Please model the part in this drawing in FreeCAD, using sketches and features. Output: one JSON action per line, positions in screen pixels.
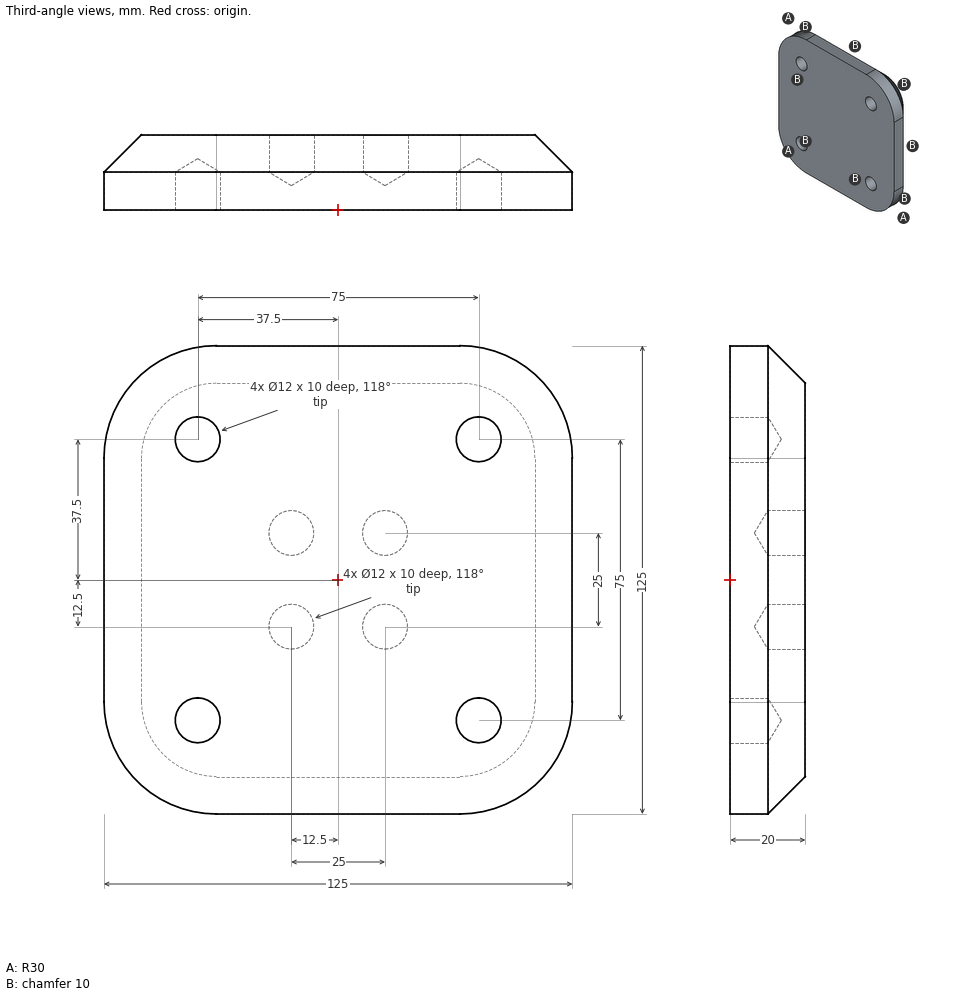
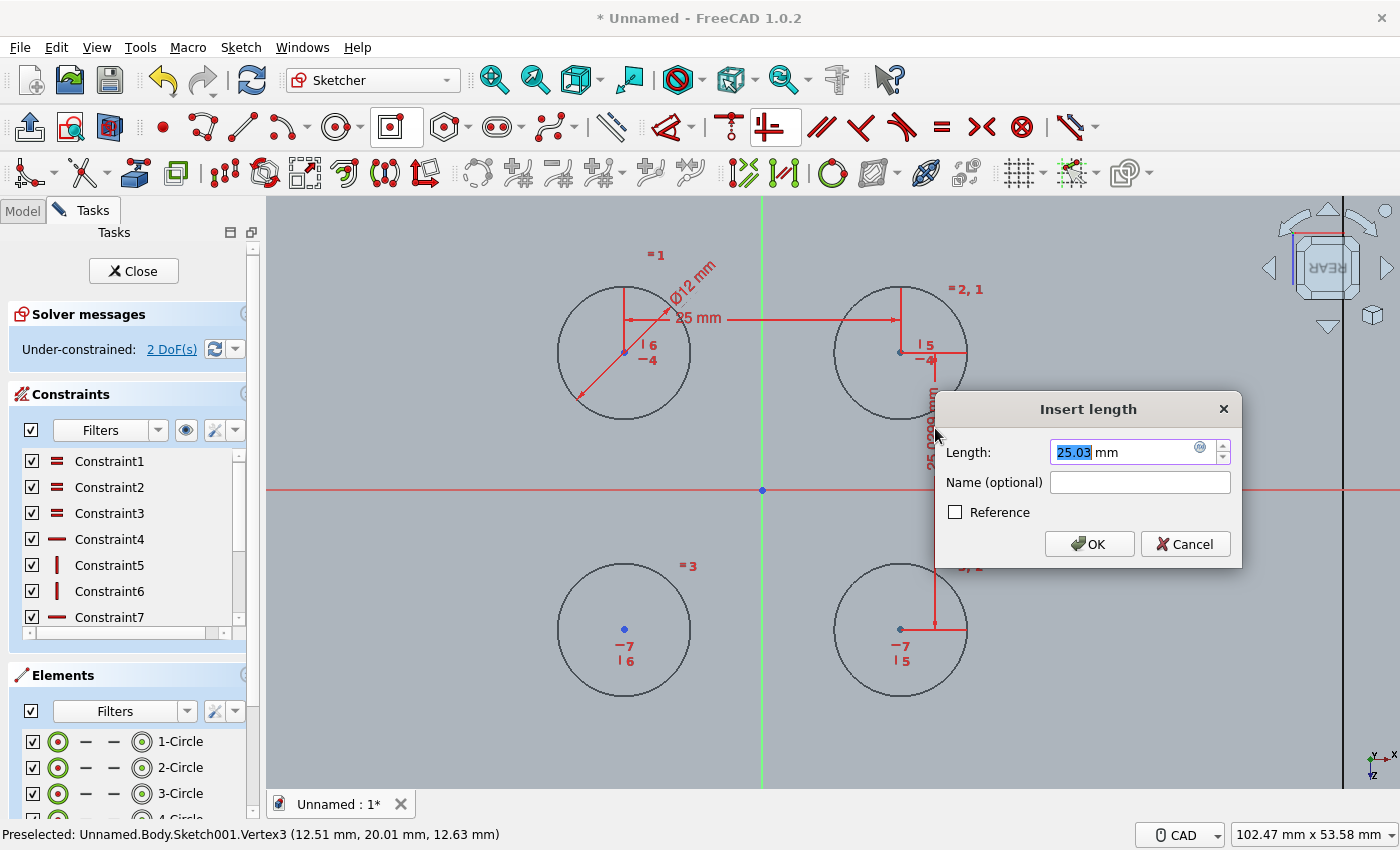
{"action": "type", "text": "25"}
{"action": "key", "text": "Return"}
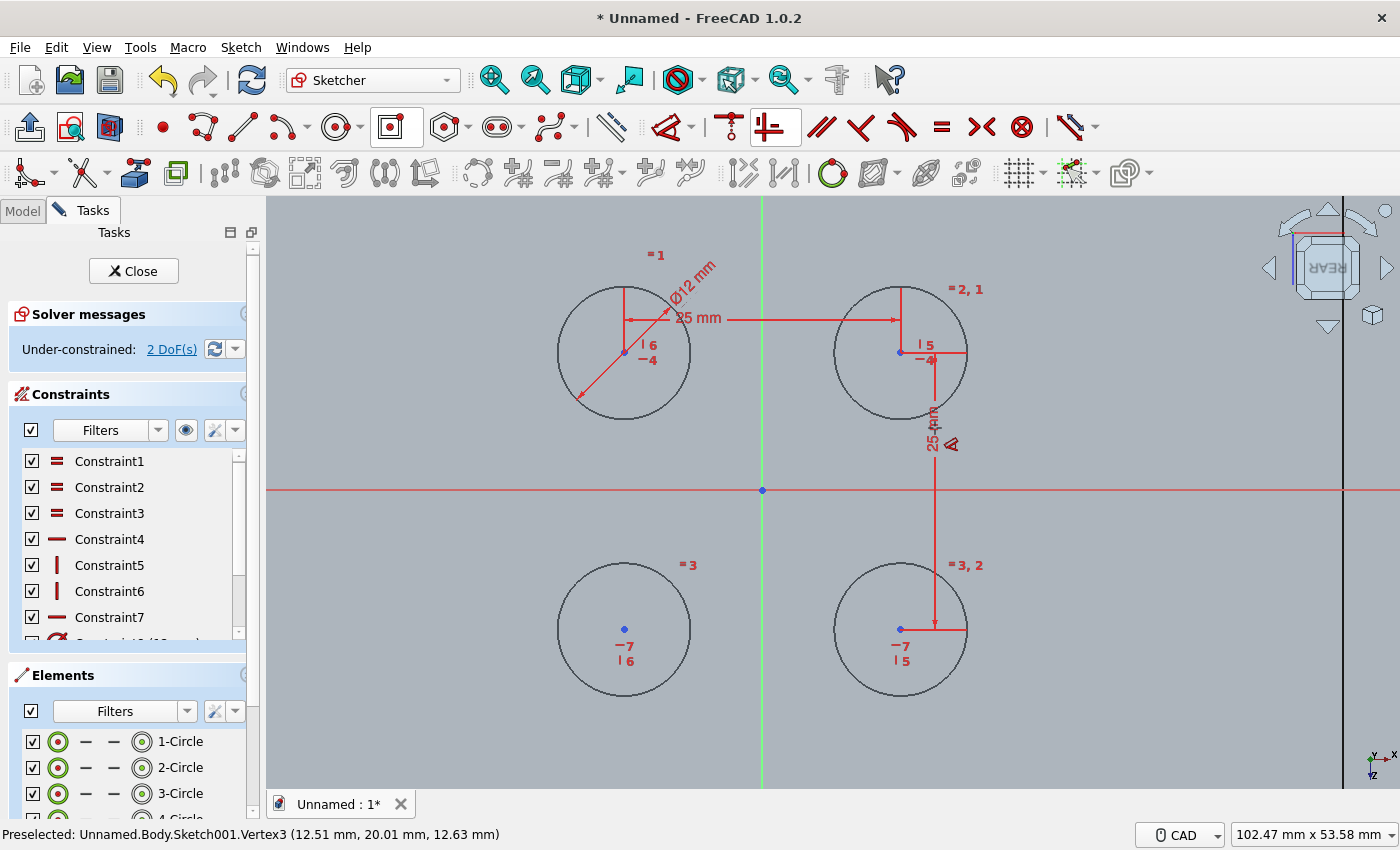
{"action": "left_click", "coordinate": [624, 353]}
{"action": "left_click", "coordinate": [693, 524]}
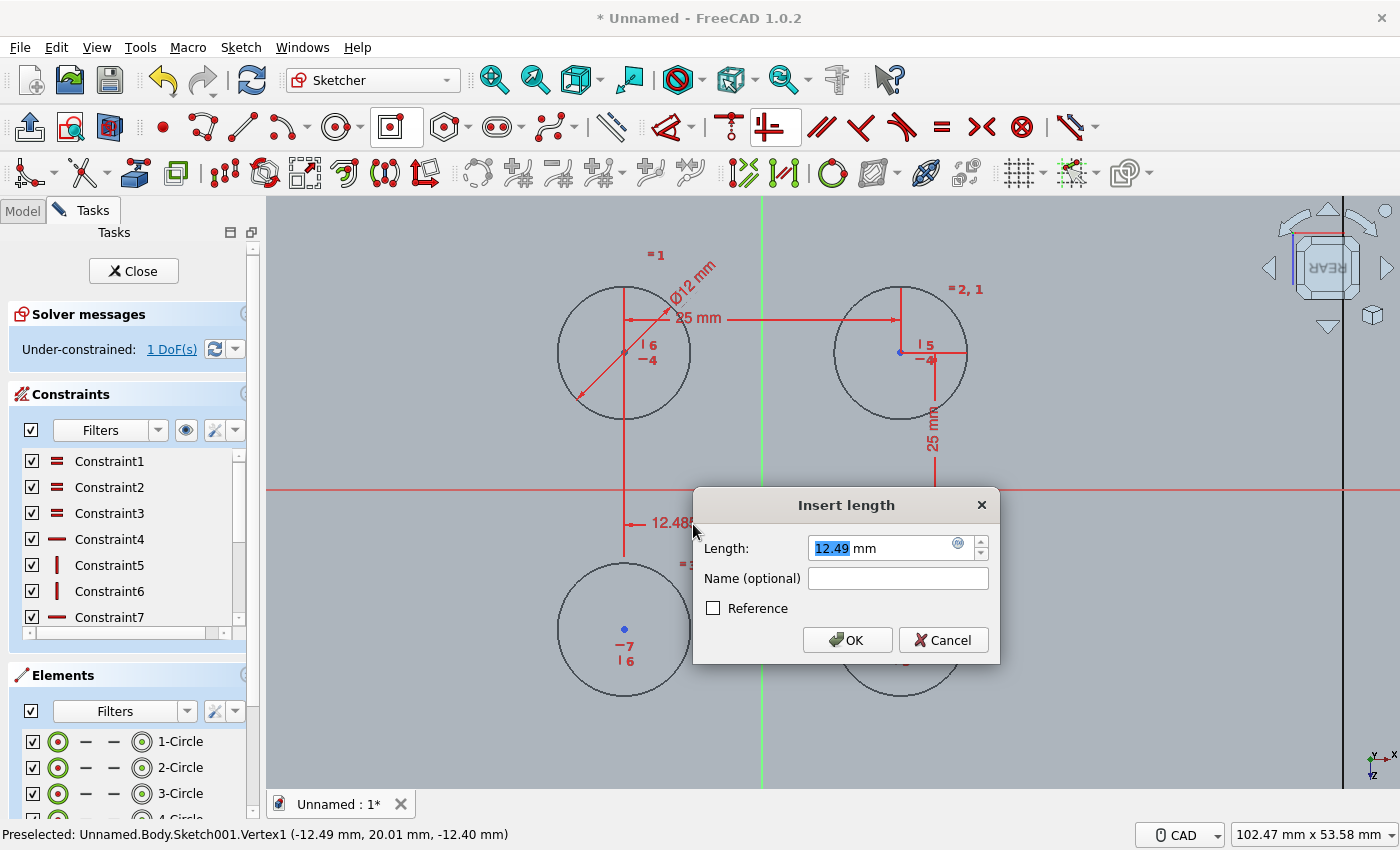
{"action": "type", "text": "12.5"}
{"action": "key", "text": "Return"}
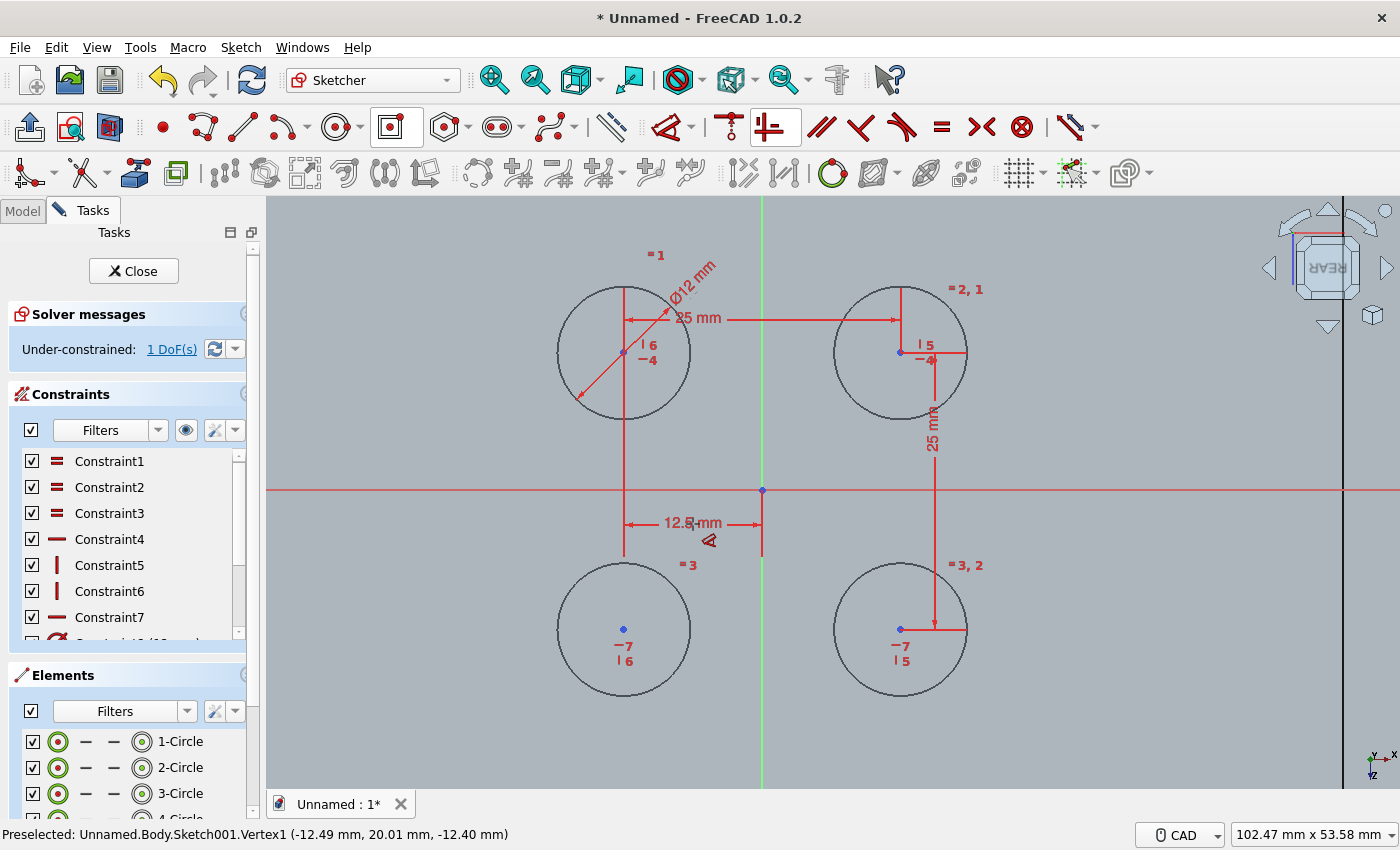
{"action": "left_click", "coordinate": [624, 353]}
{"action": "left_click", "coordinate": [590, 390]}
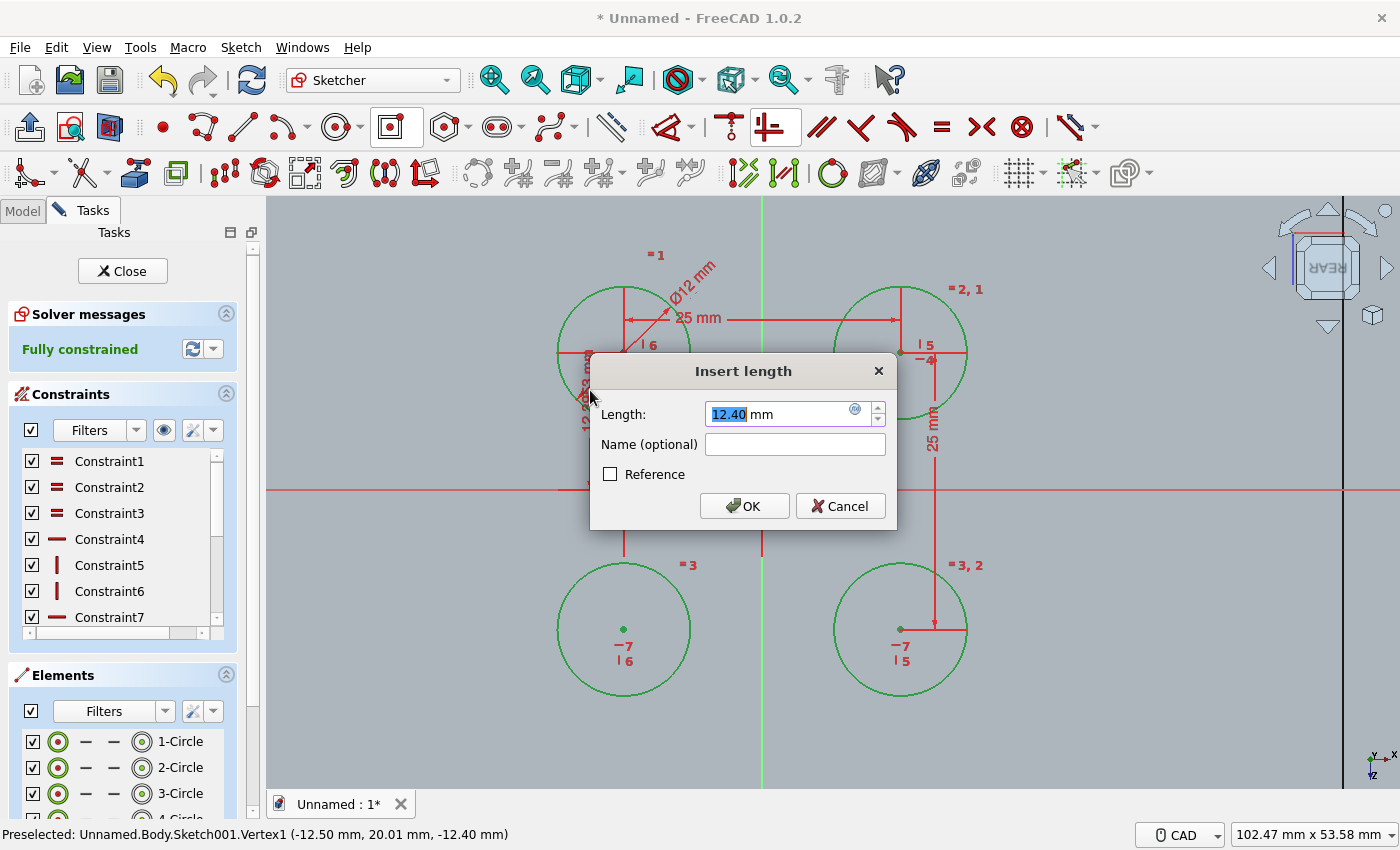
{"action": "type", "text": "12.5"}
{"action": "key", "text": "Return"}
{"action": "key", "text": "Escape"}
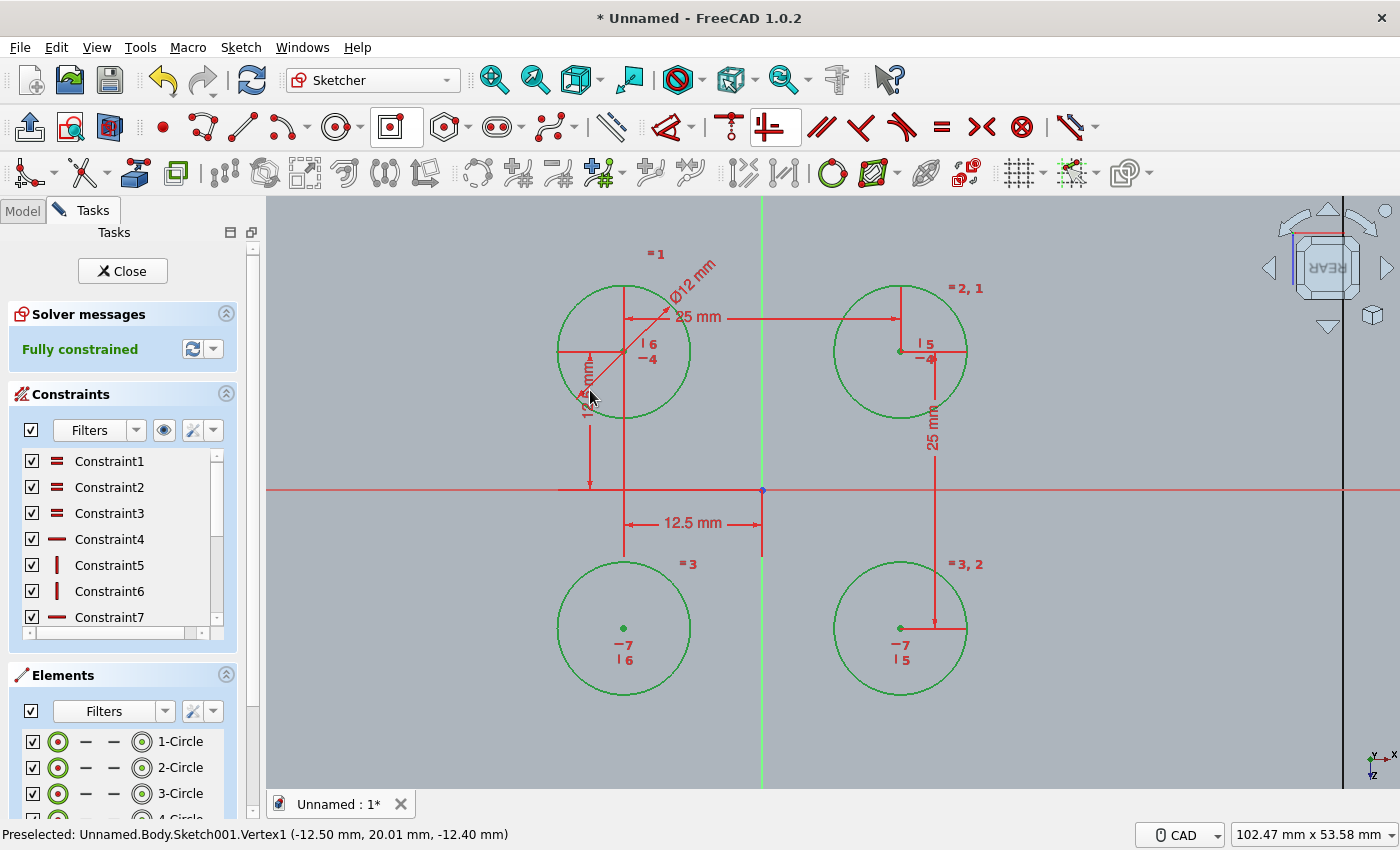
{"action": "left_click", "coordinate": [123, 271]}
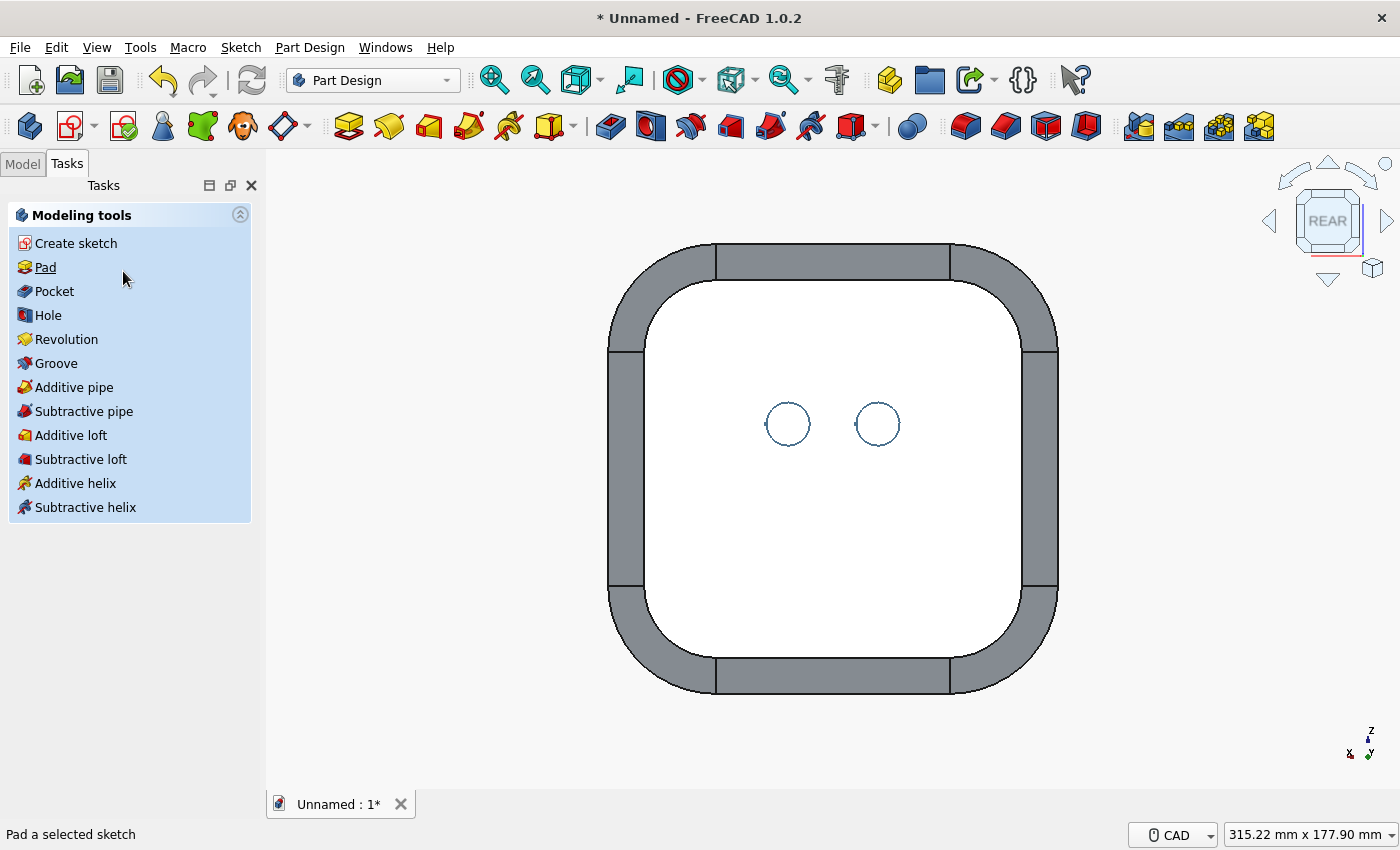
{"action": "left_click", "coordinate": [652, 126]}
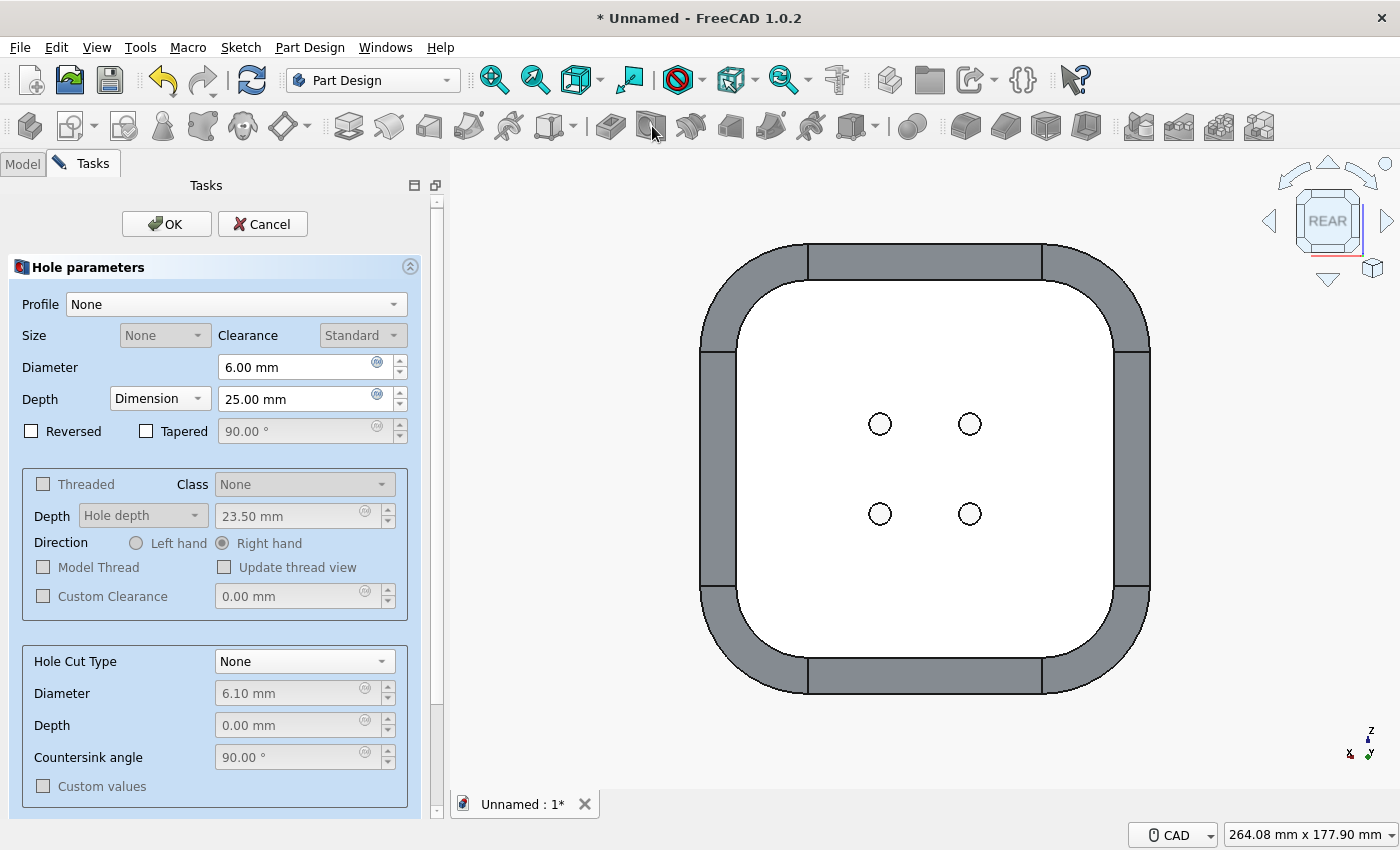
{"action": "triple_click", "coordinate": [305, 367]}